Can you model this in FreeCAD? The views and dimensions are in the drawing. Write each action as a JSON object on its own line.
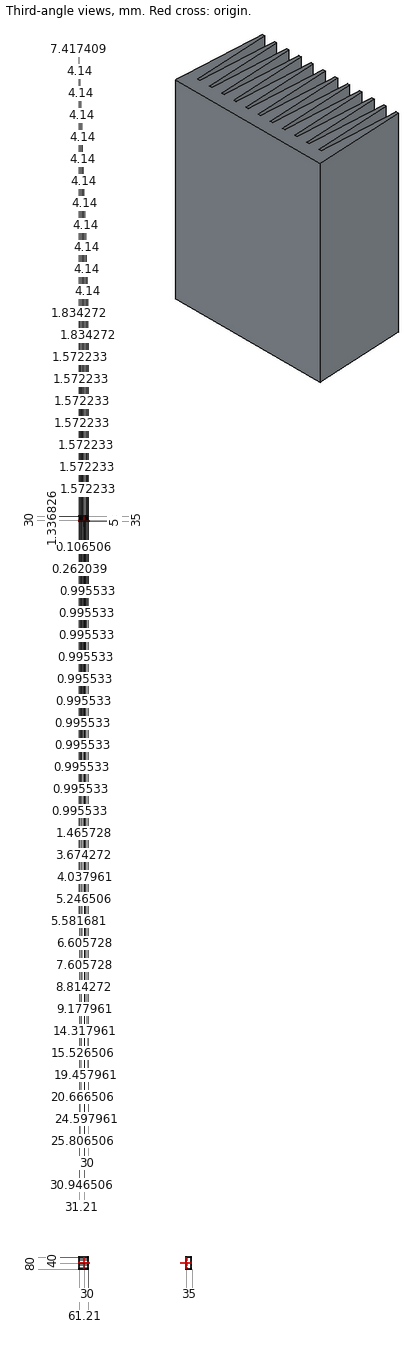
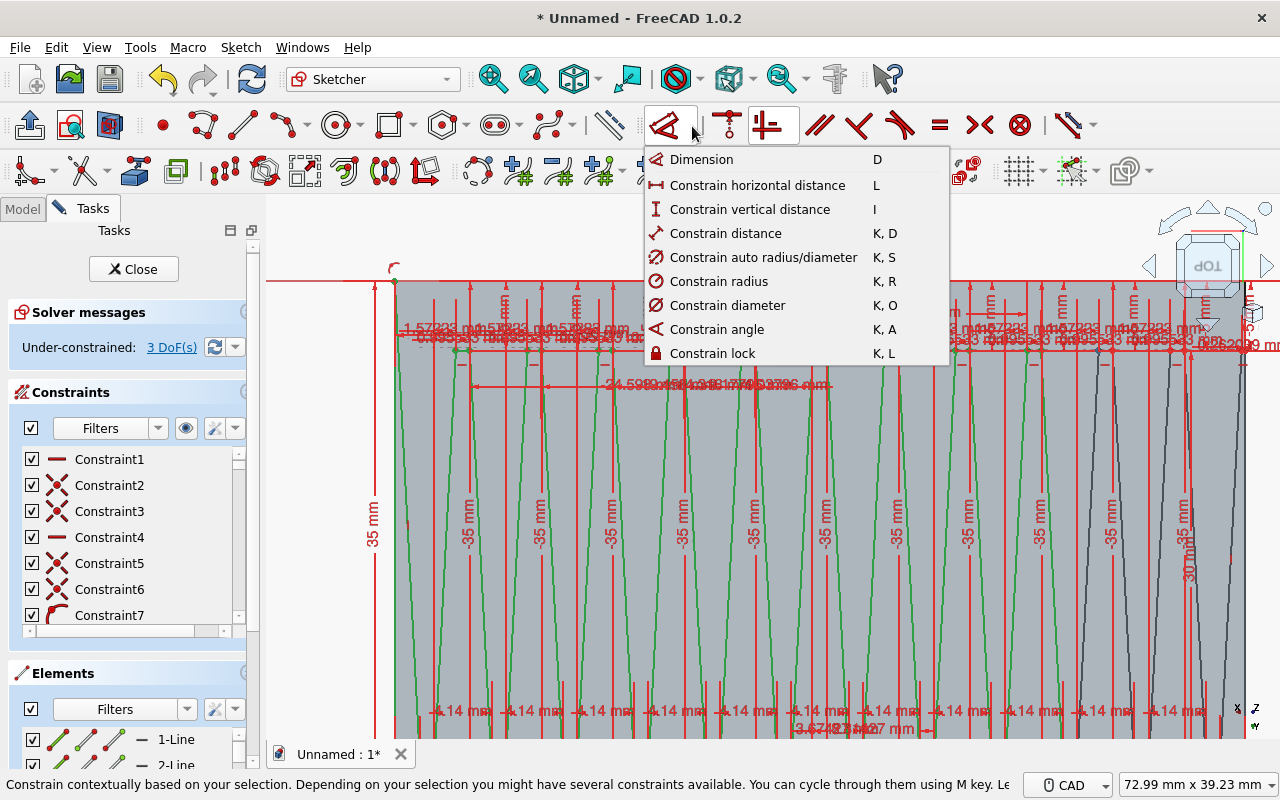
{"action": "left_click", "coordinate": [797, 185]}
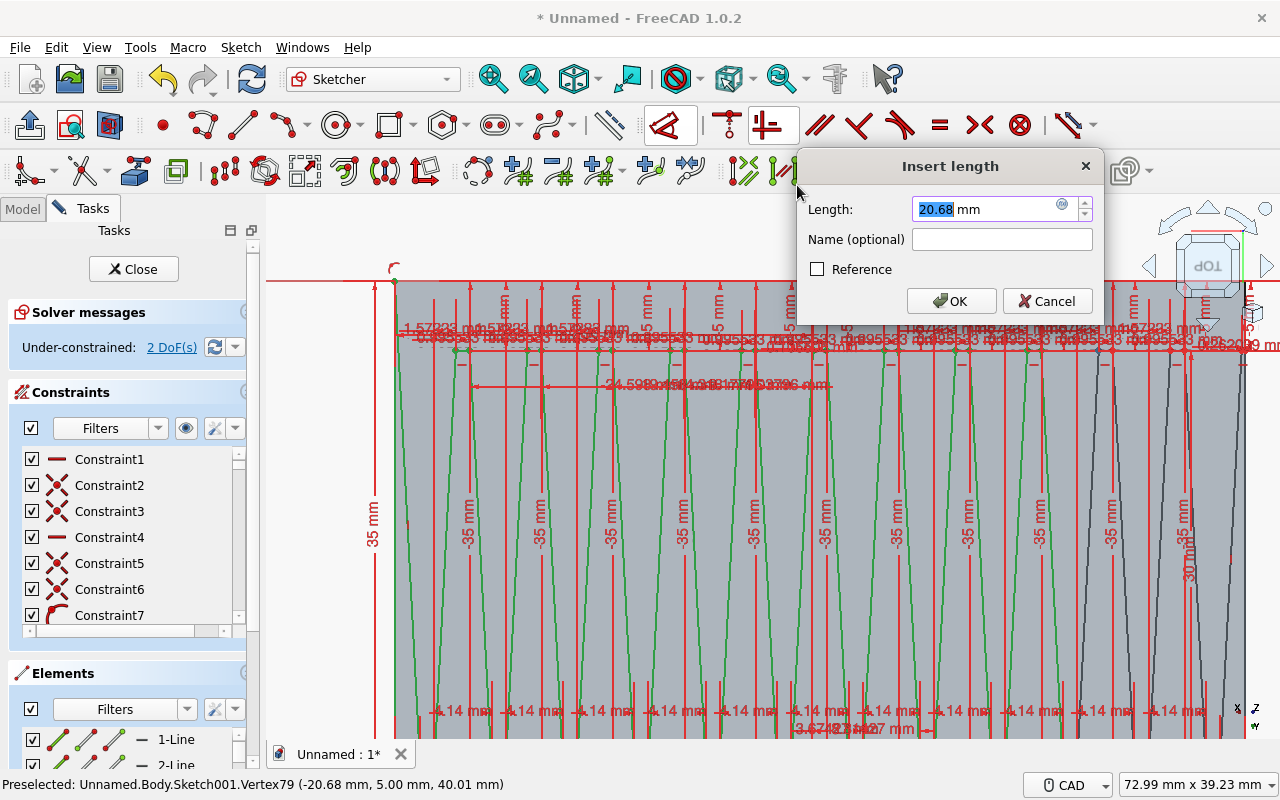
{"action": "type", "text": "20.666506"}
{"action": "key", "text": "Return"}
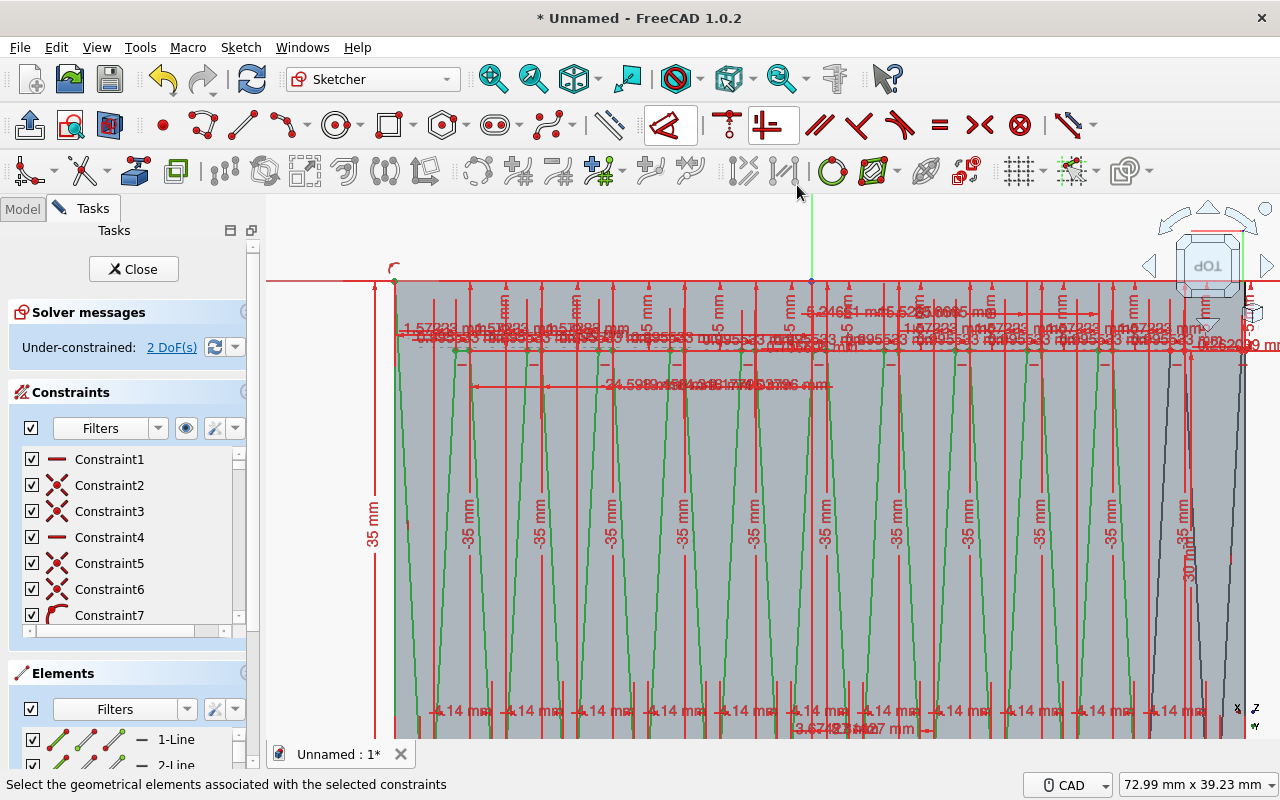
{"action": "scroll", "coordinate": [470, 349], "scroll_direction": "down", "scroll_amount": 2}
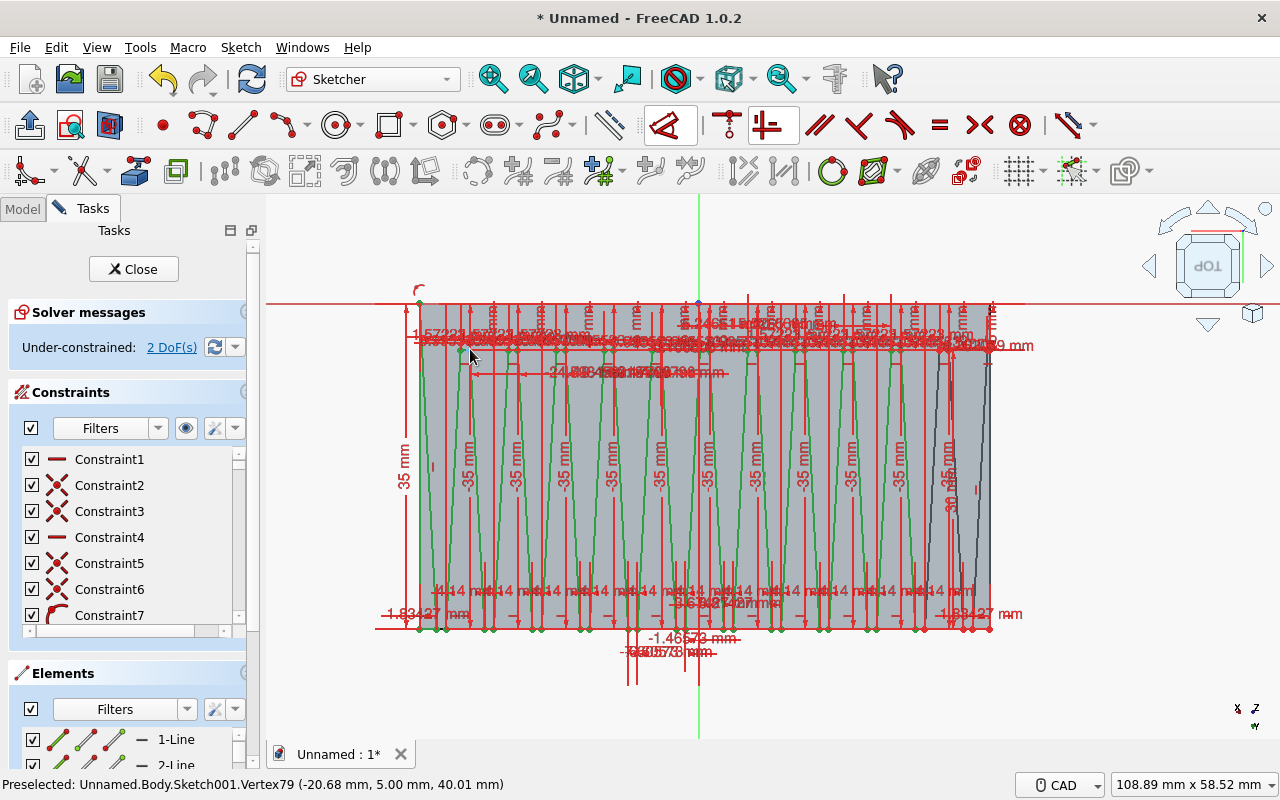
{"action": "scroll", "coordinate": [940, 350], "scroll_direction": "up", "scroll_amount": 2}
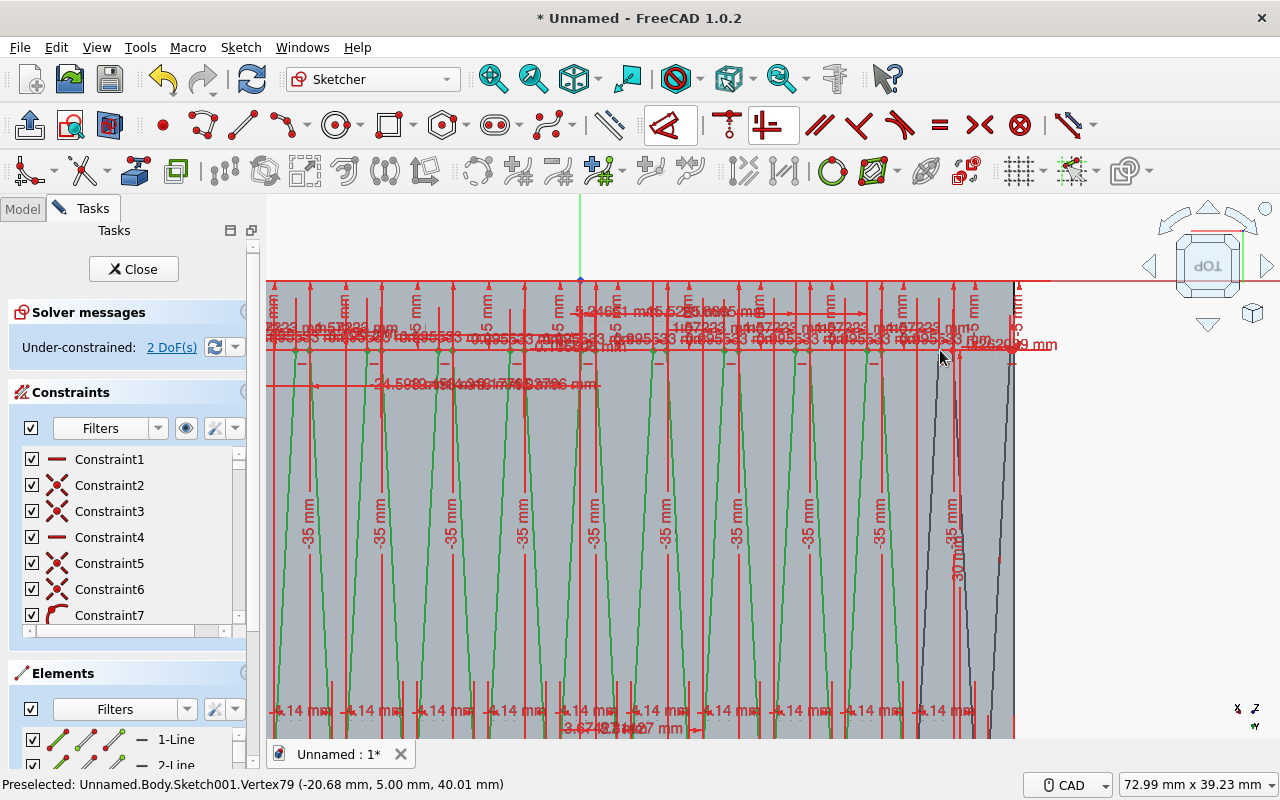
{"action": "left_click", "coordinate": [939, 350]}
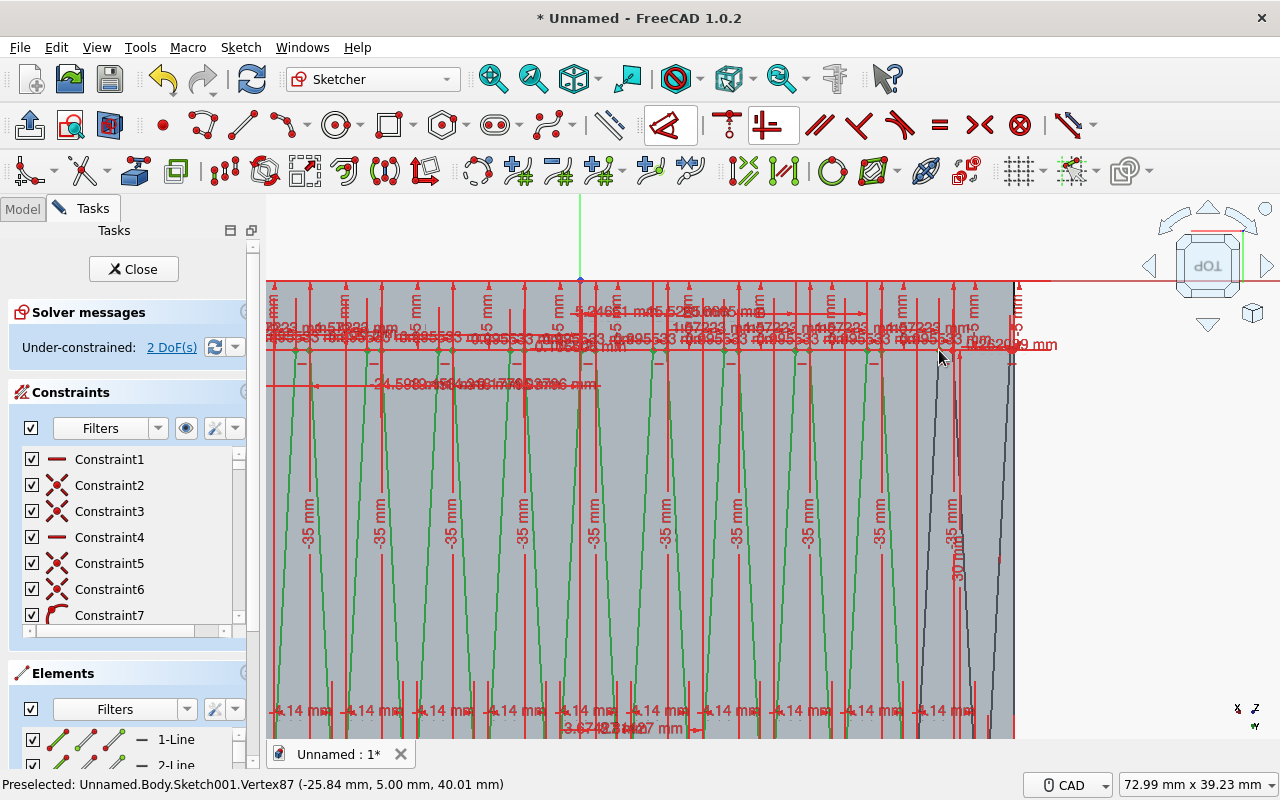
{"action": "key", "text": "l"}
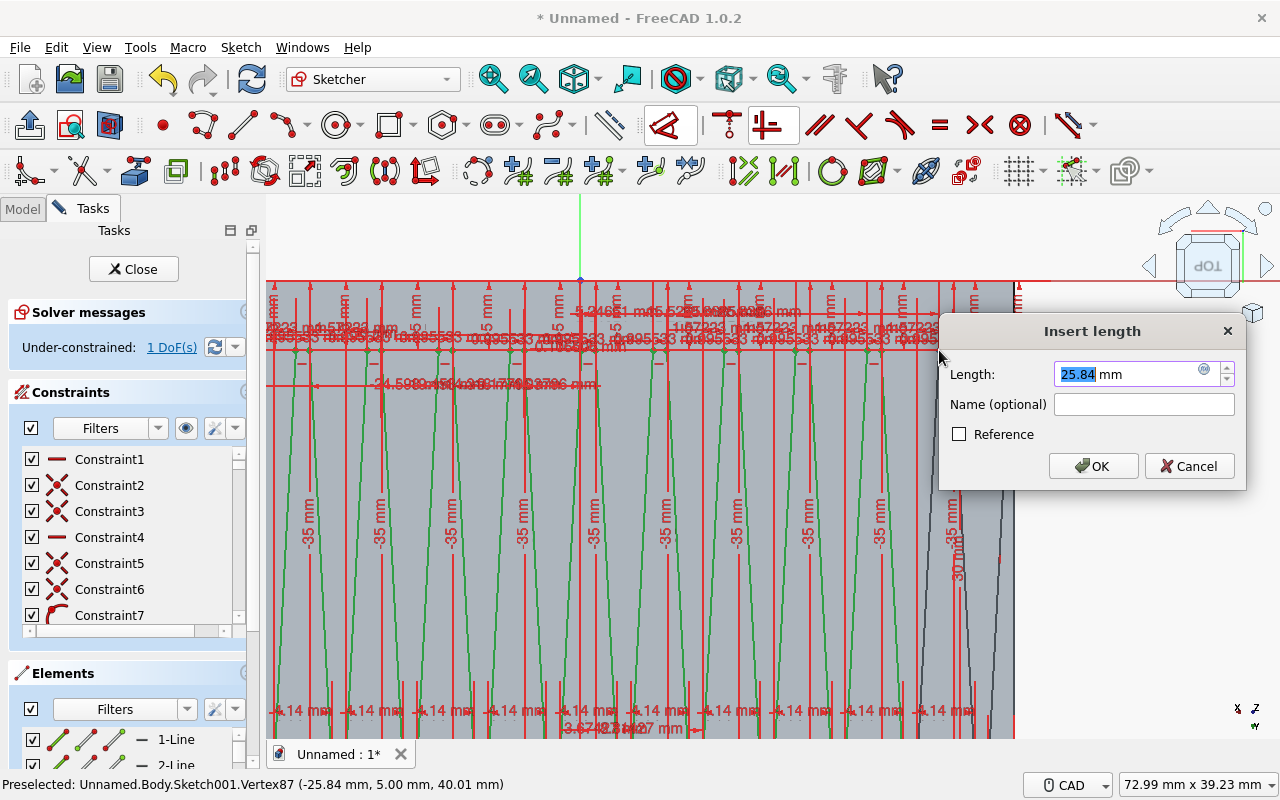
{"action": "type", "text": "25.806506"}
{"action": "key", "text": "Return"}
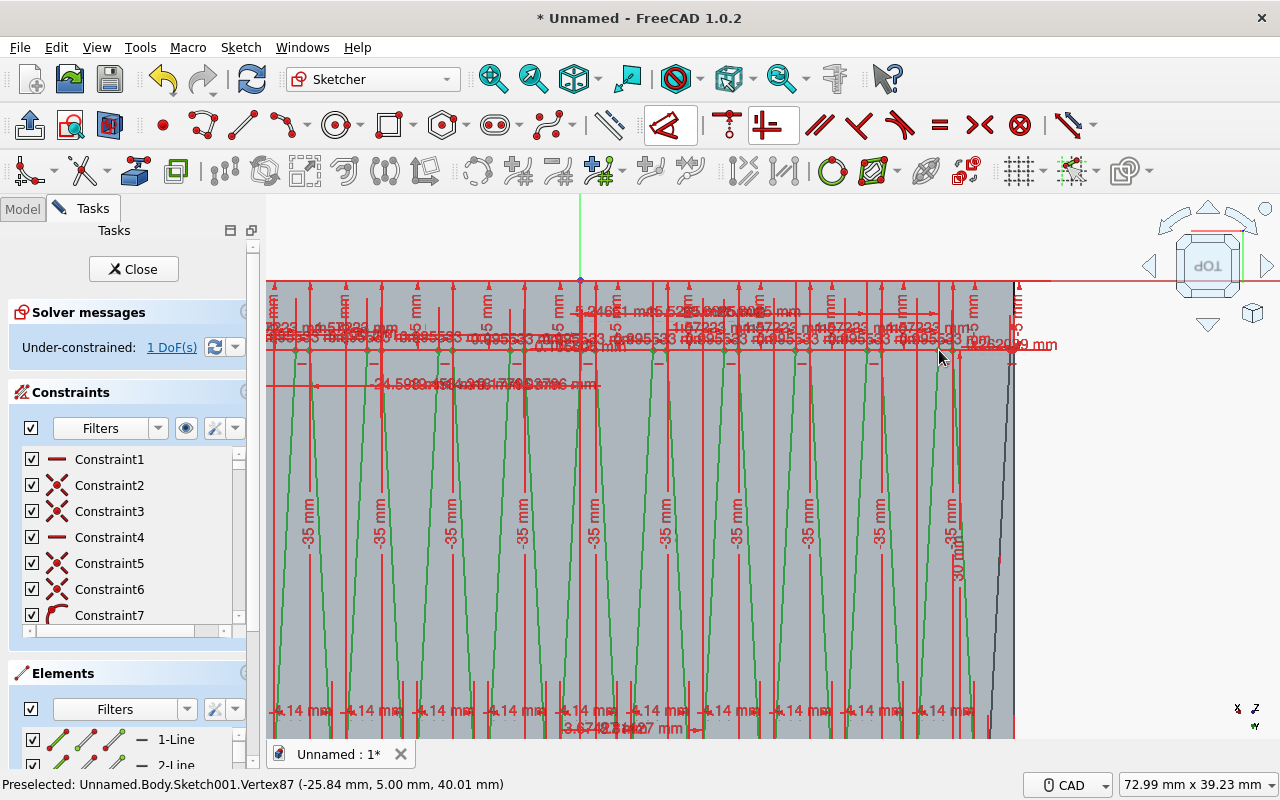
{"action": "scroll", "coordinate": [1010, 350], "scroll_direction": "up", "scroll_amount": 7}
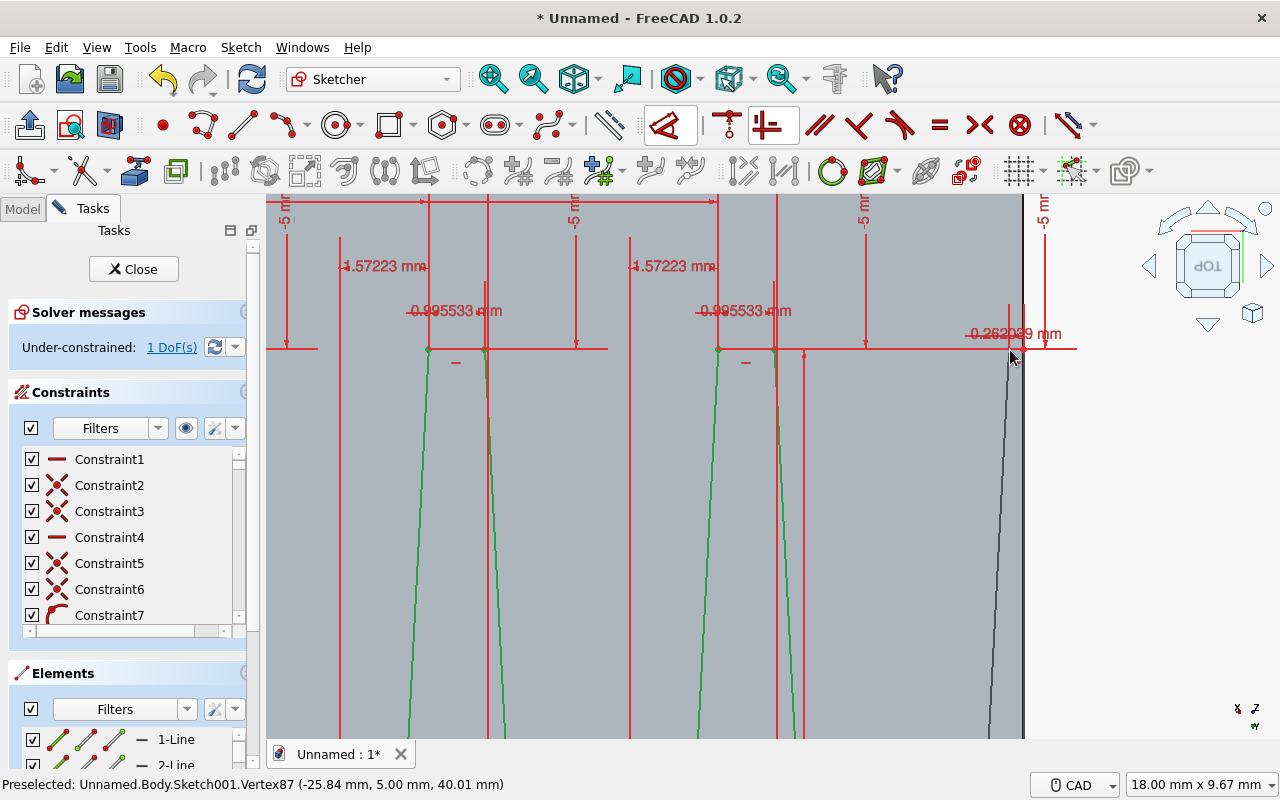
{"action": "left_click", "coordinate": [1009, 349]}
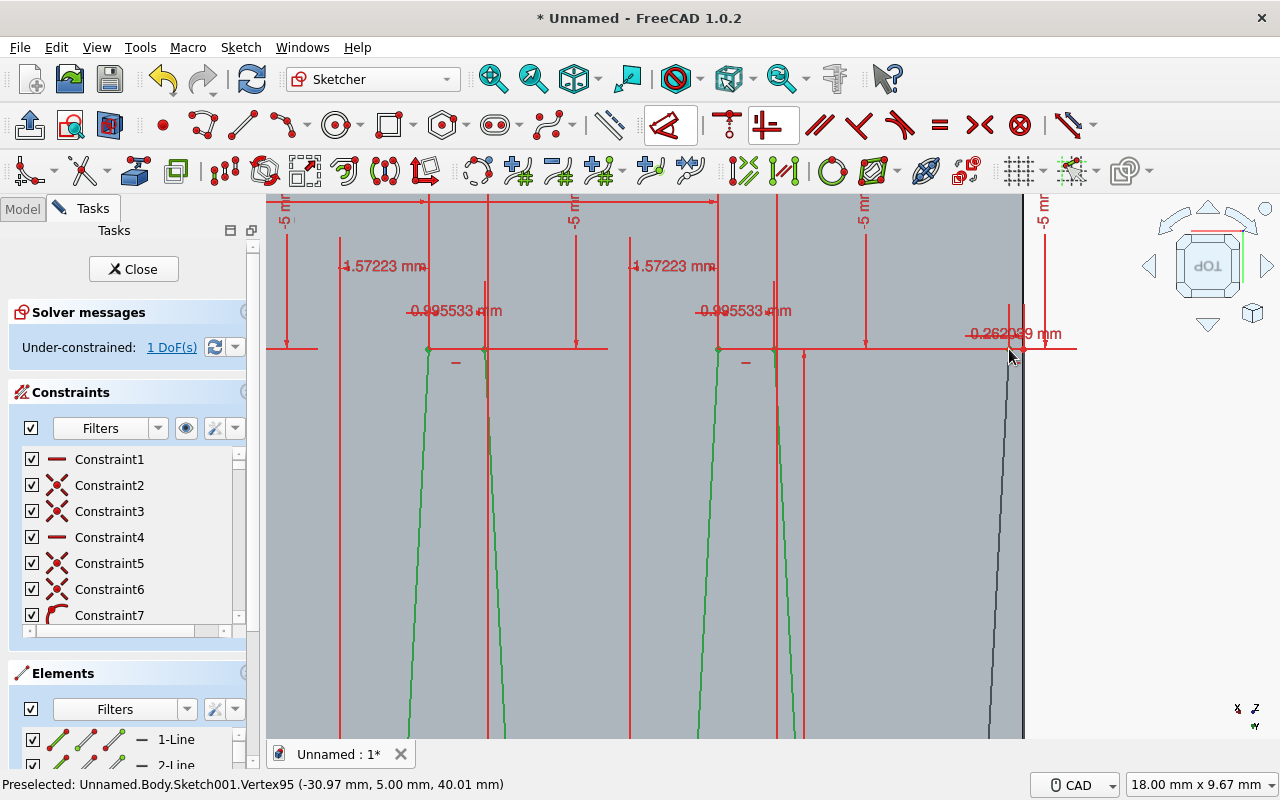
{"action": "key", "text": "l"}